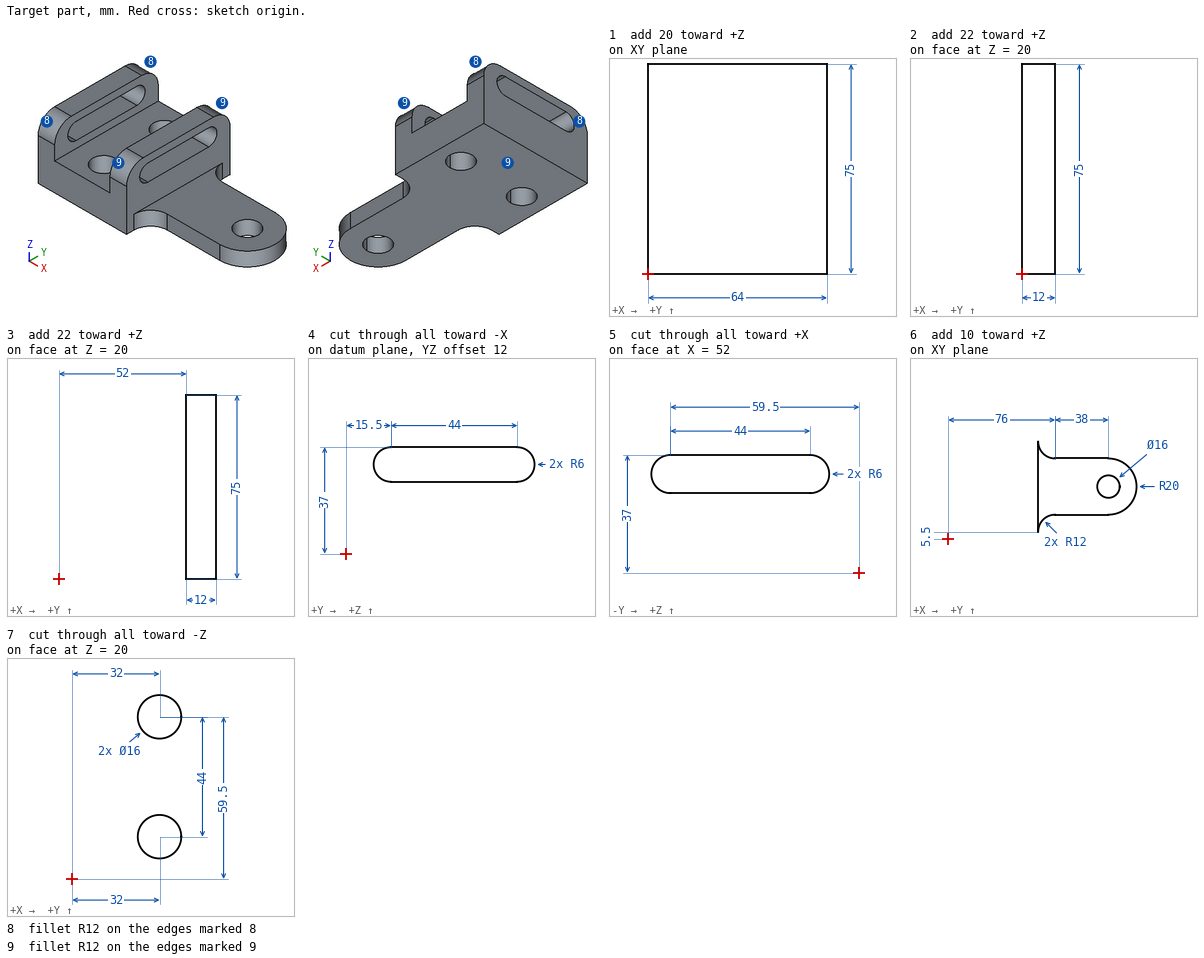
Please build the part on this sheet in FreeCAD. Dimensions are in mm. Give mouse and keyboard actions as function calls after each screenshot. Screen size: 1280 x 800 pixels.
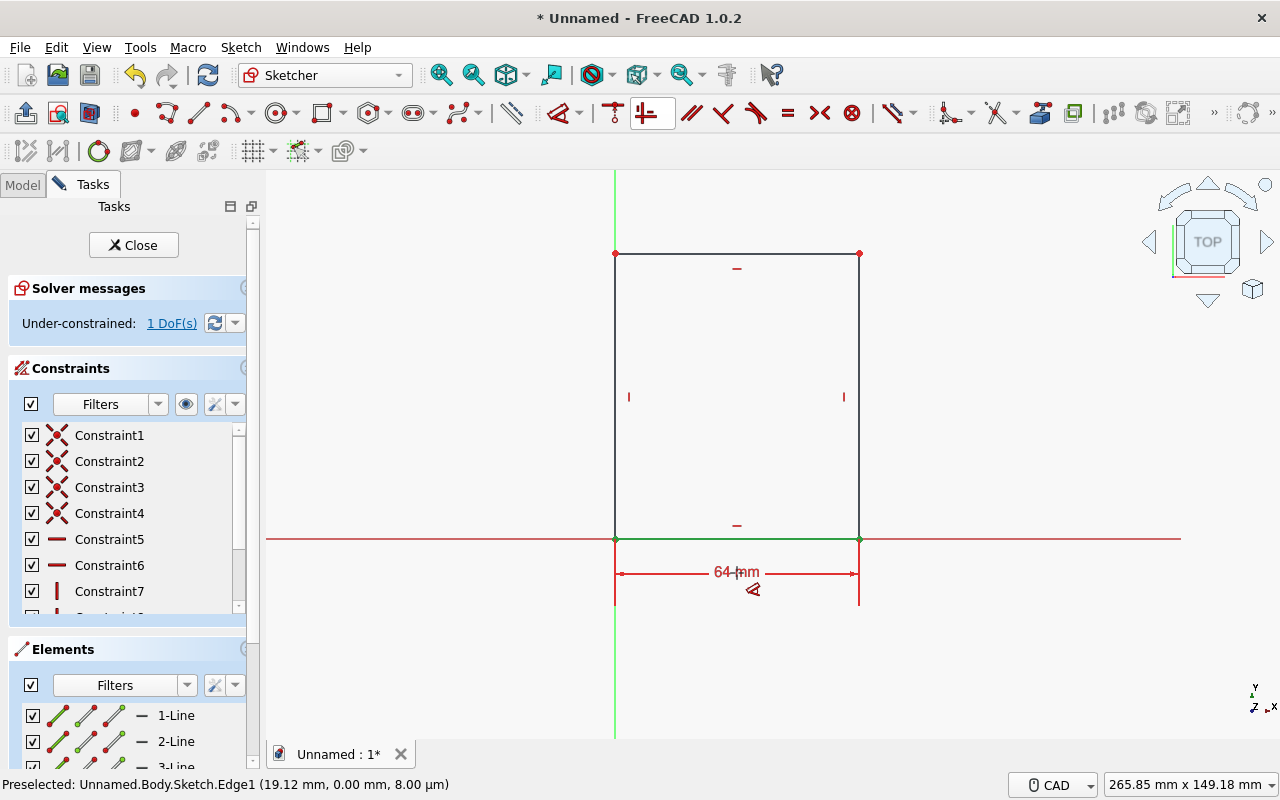
click(859, 454)
click(893, 397)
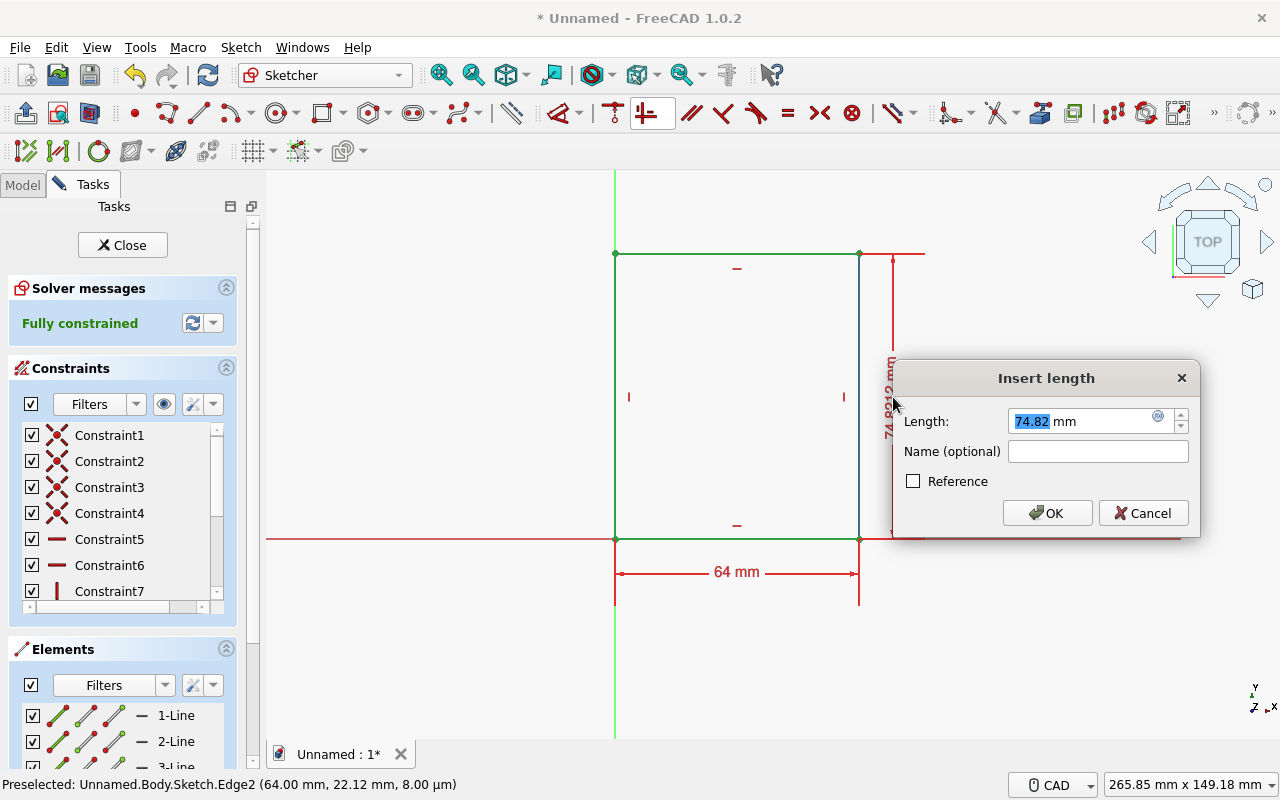
text(75)
key(Return)
key(Escape)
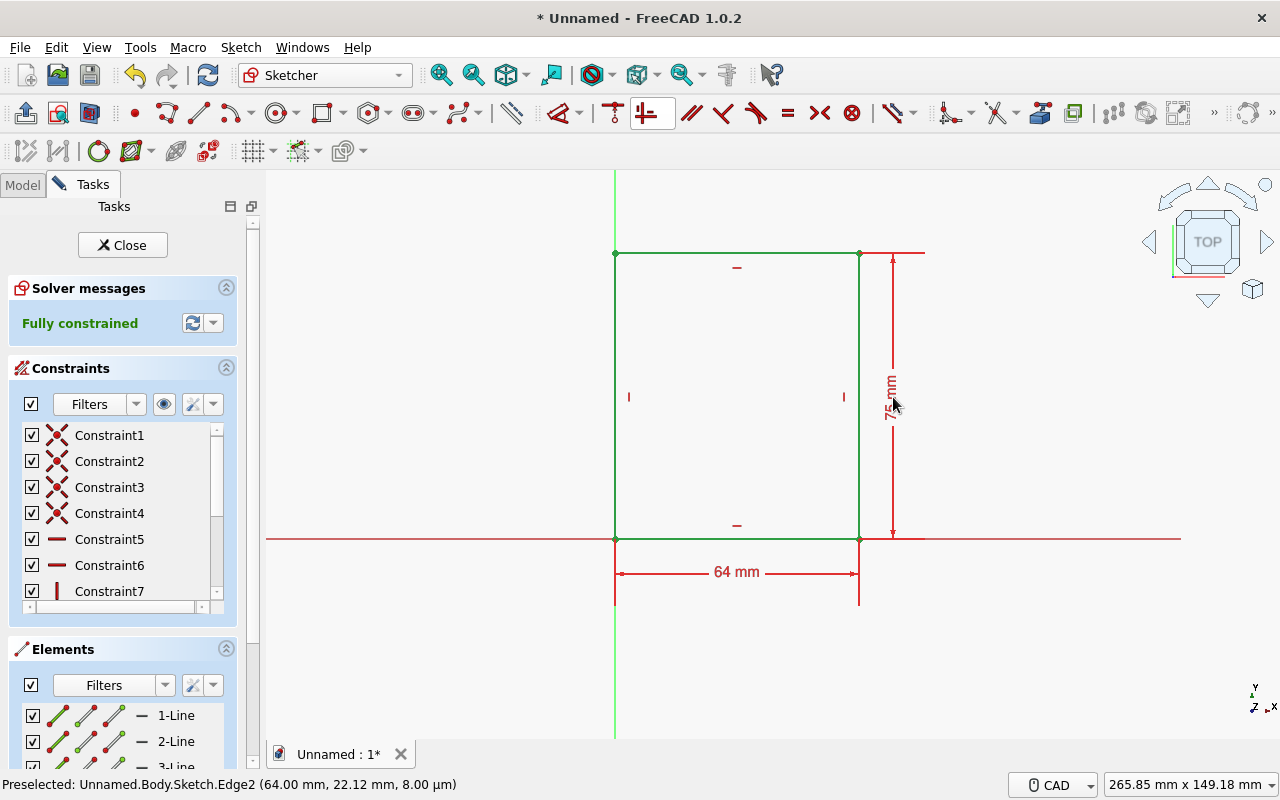
click(123, 245)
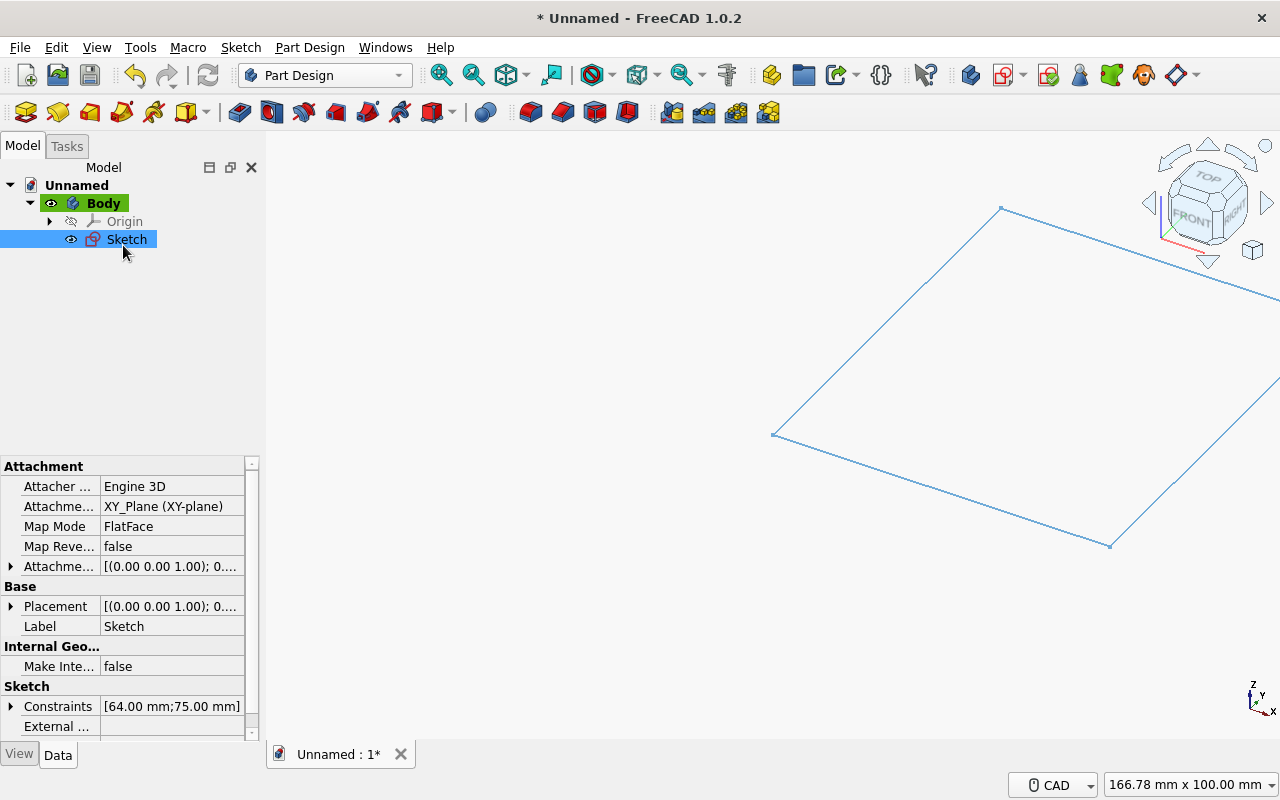
click(26, 112)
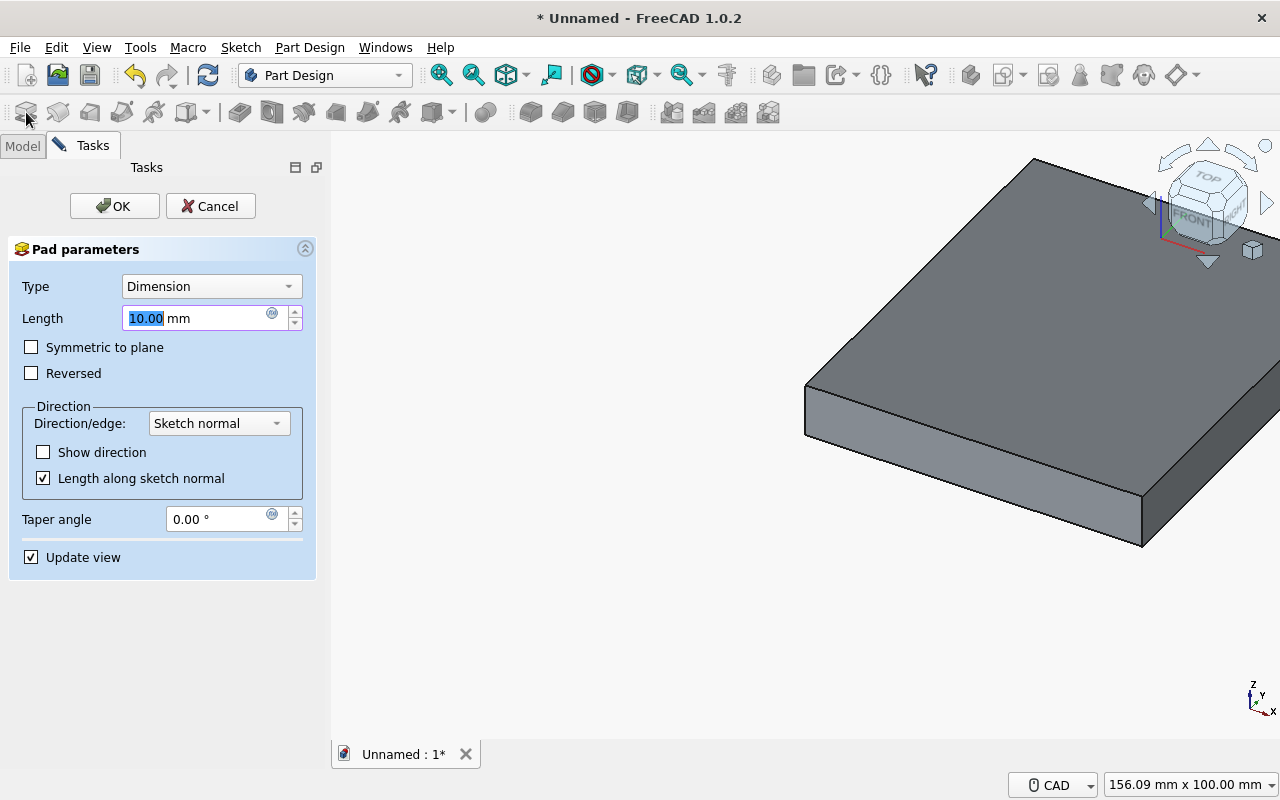
text(20)
key(Tab)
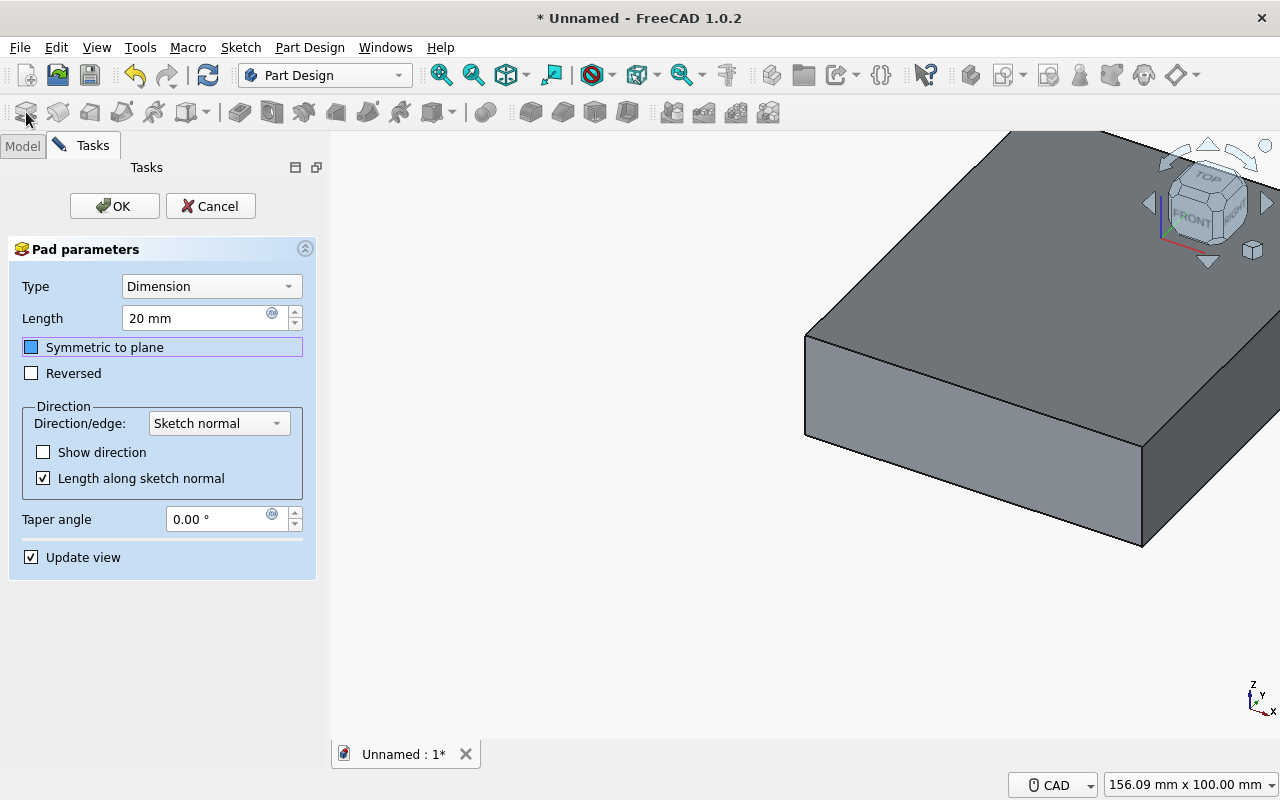
click(115, 206)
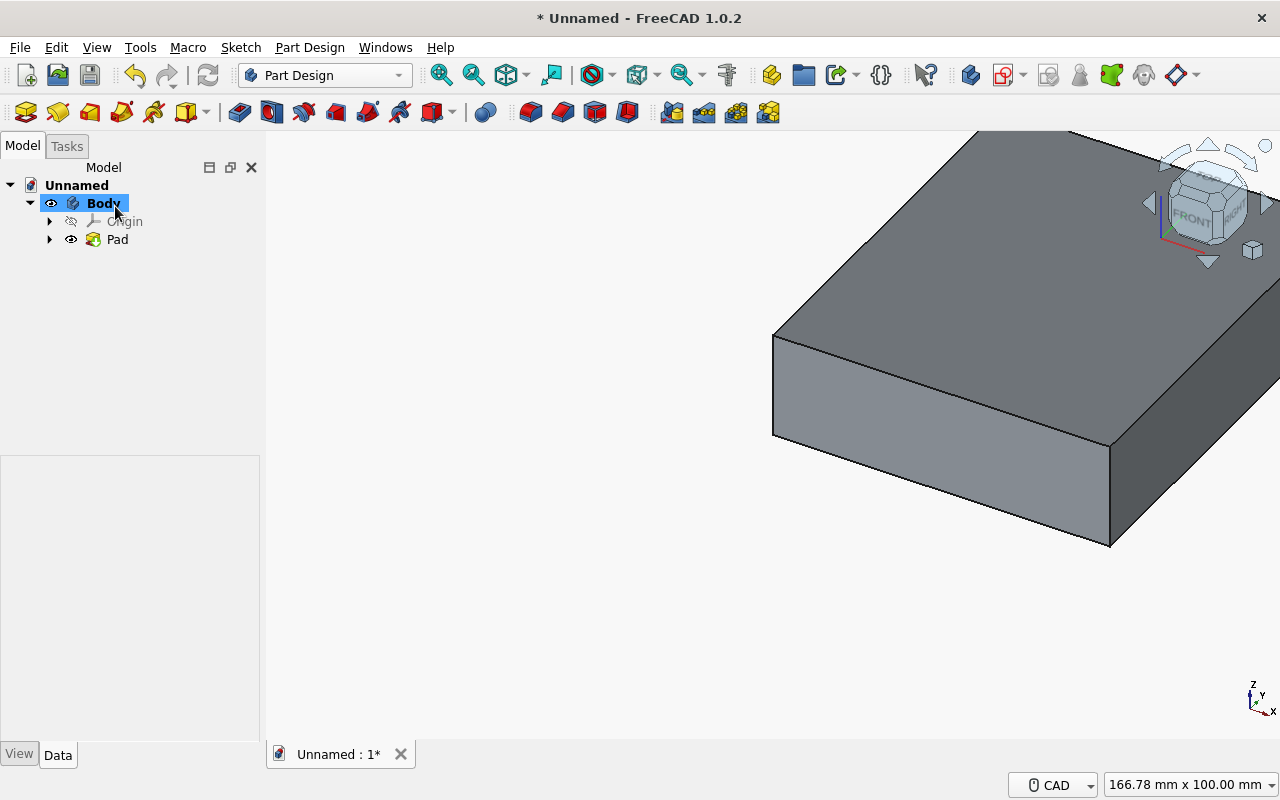
click(442, 76)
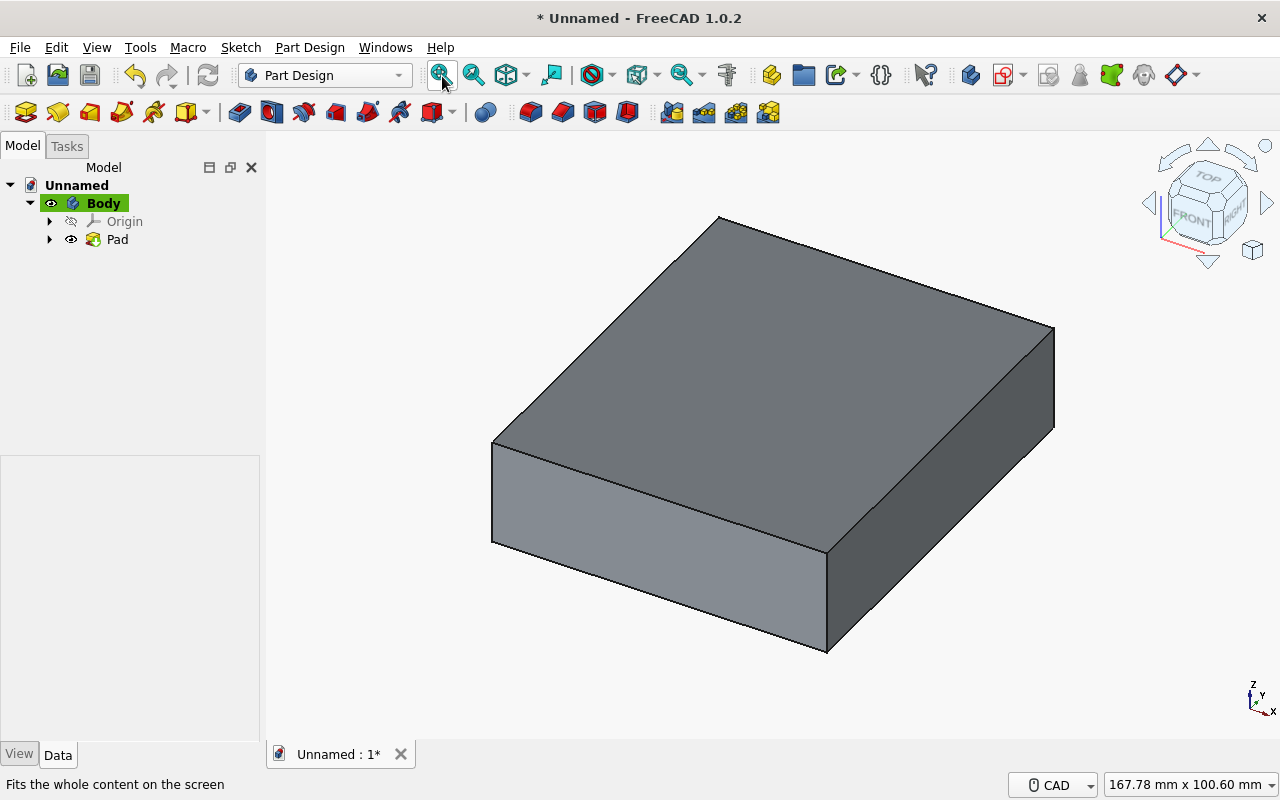
click(773, 384)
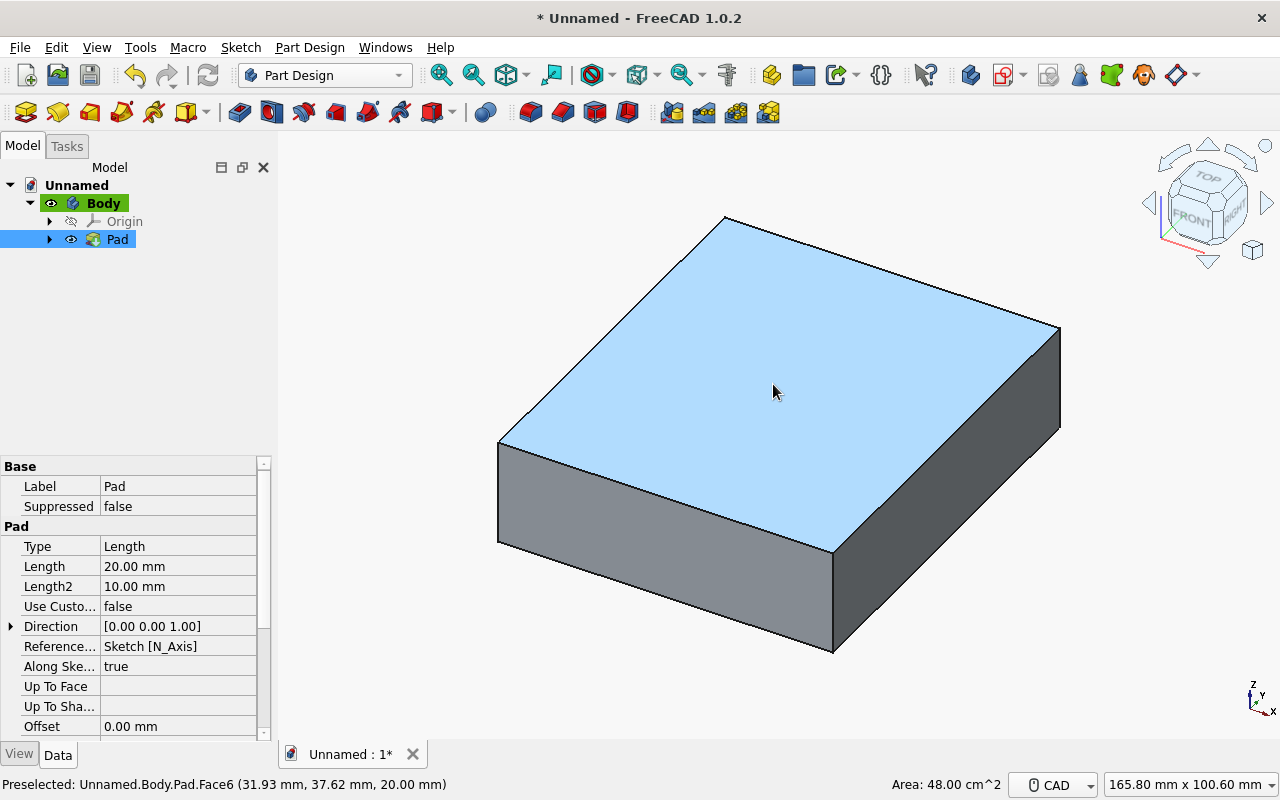
click(1004, 76)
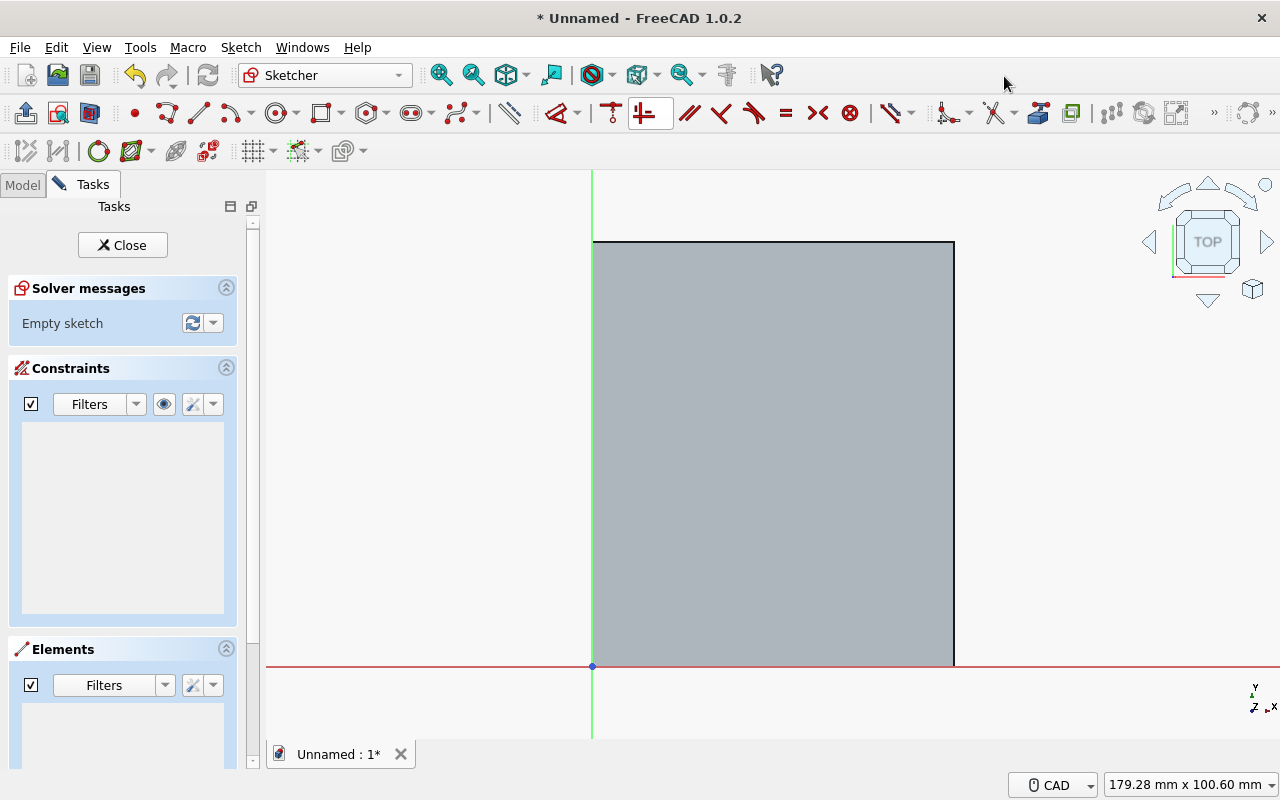
click(322, 114)